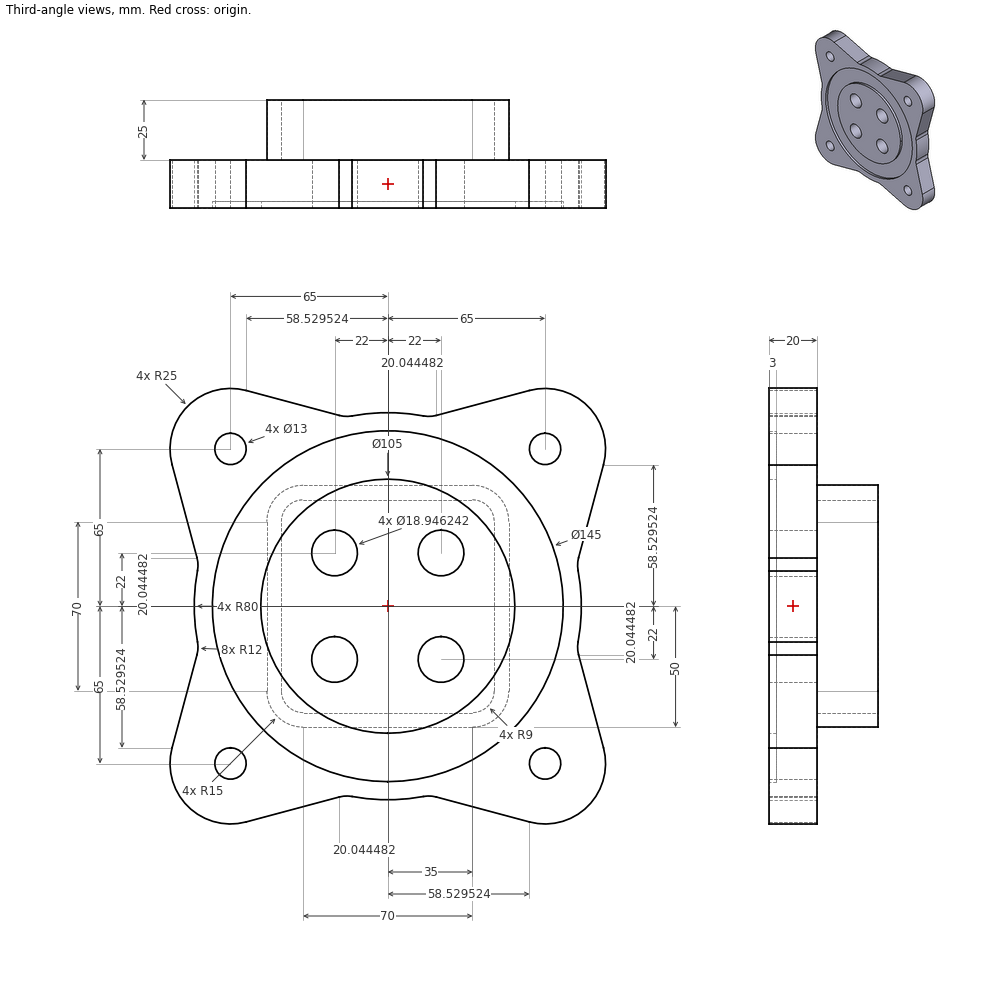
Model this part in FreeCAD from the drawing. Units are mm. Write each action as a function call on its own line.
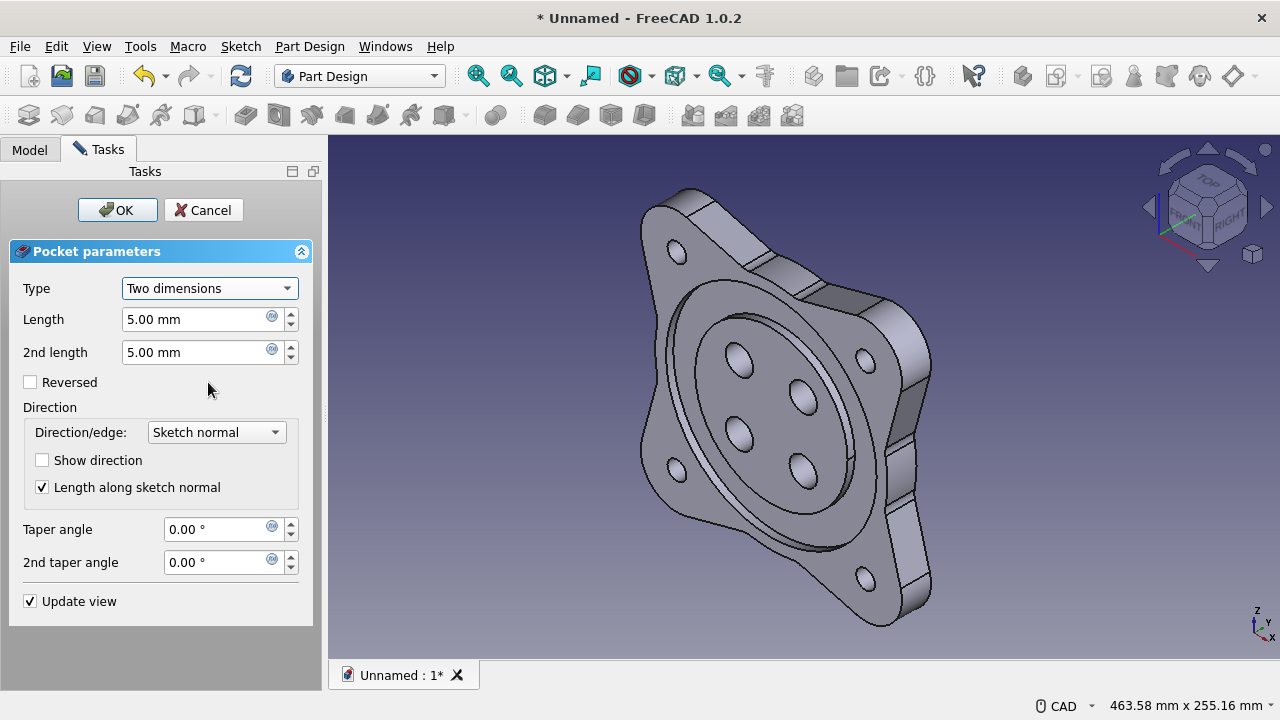
triple_click(204, 320)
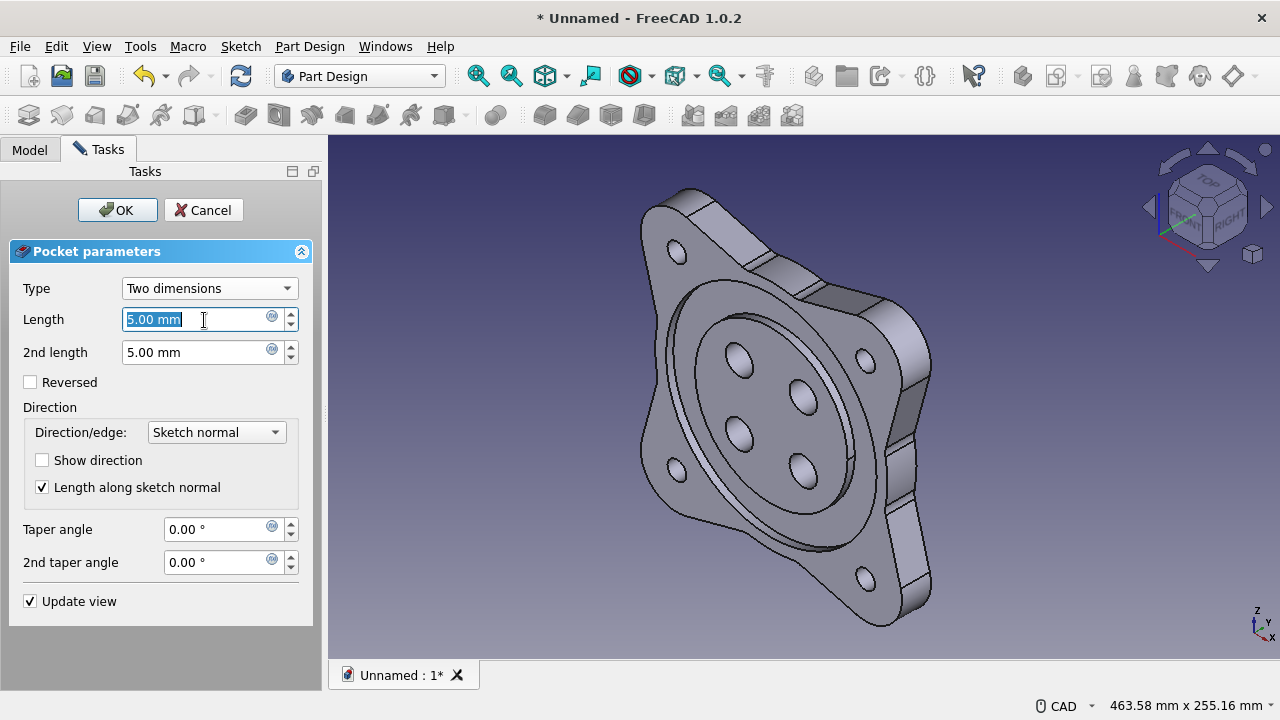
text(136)
key(Tab)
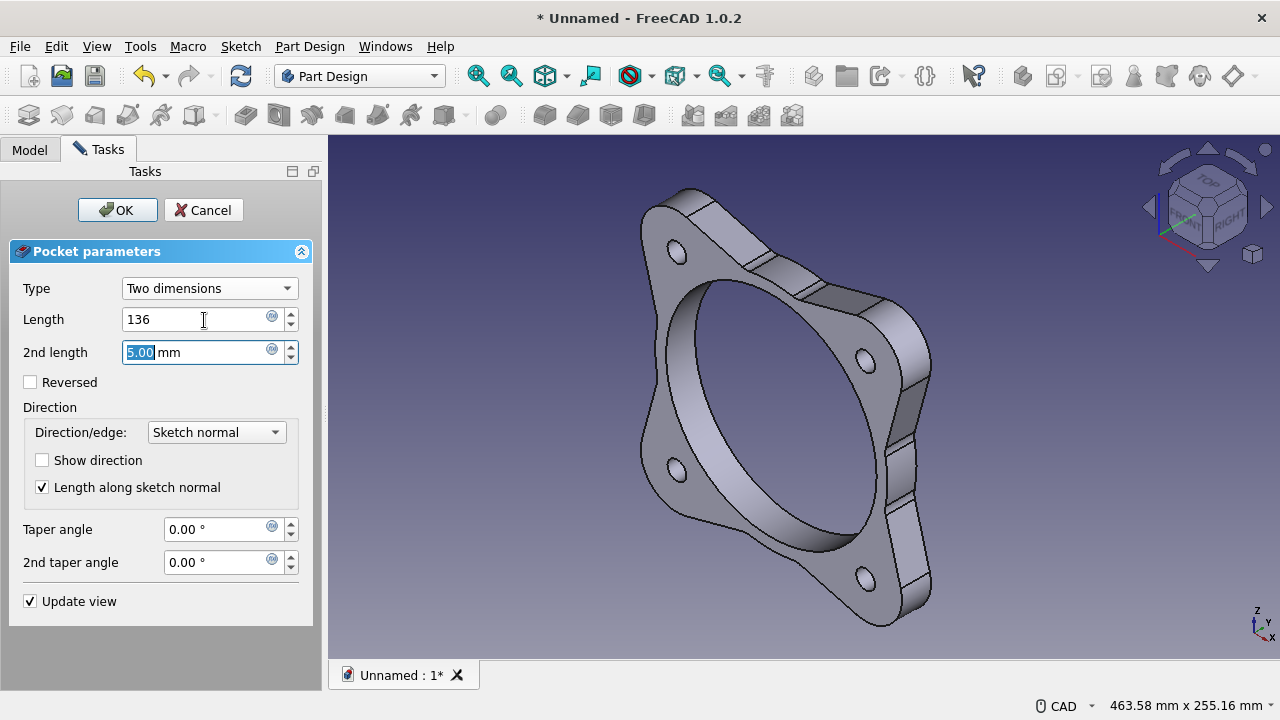
text(3)
key(Tab)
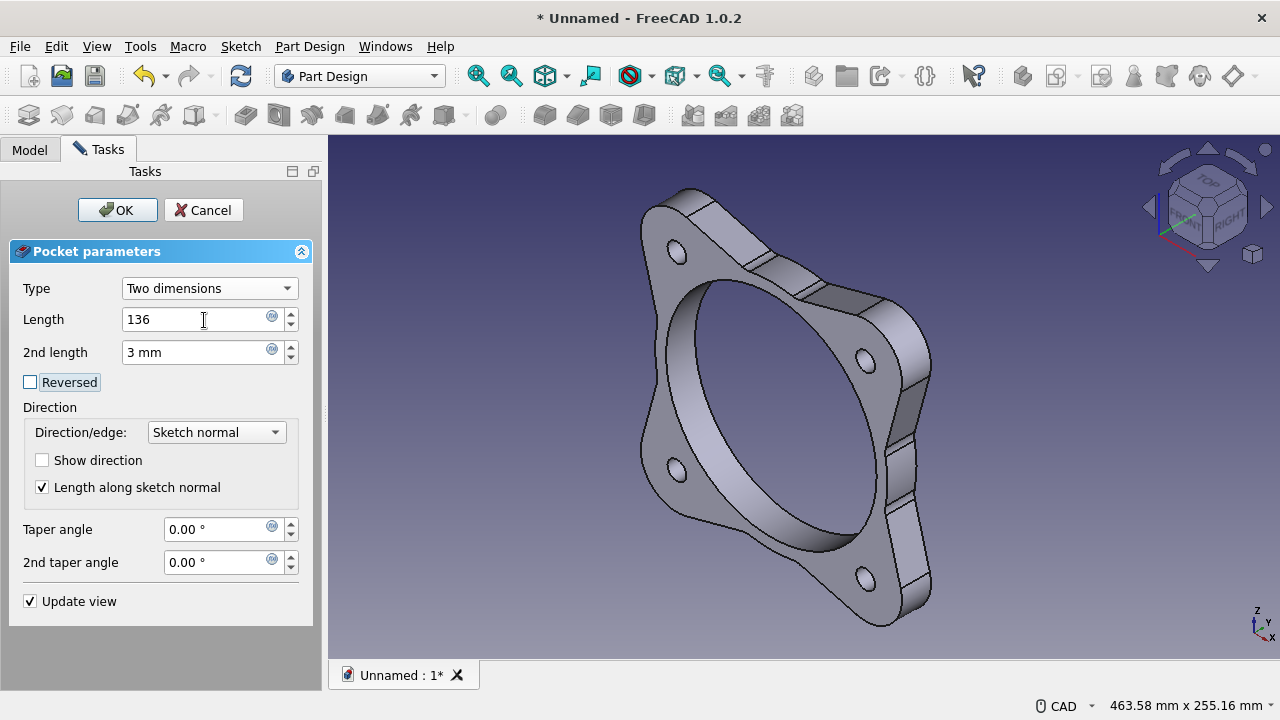
click(31, 382)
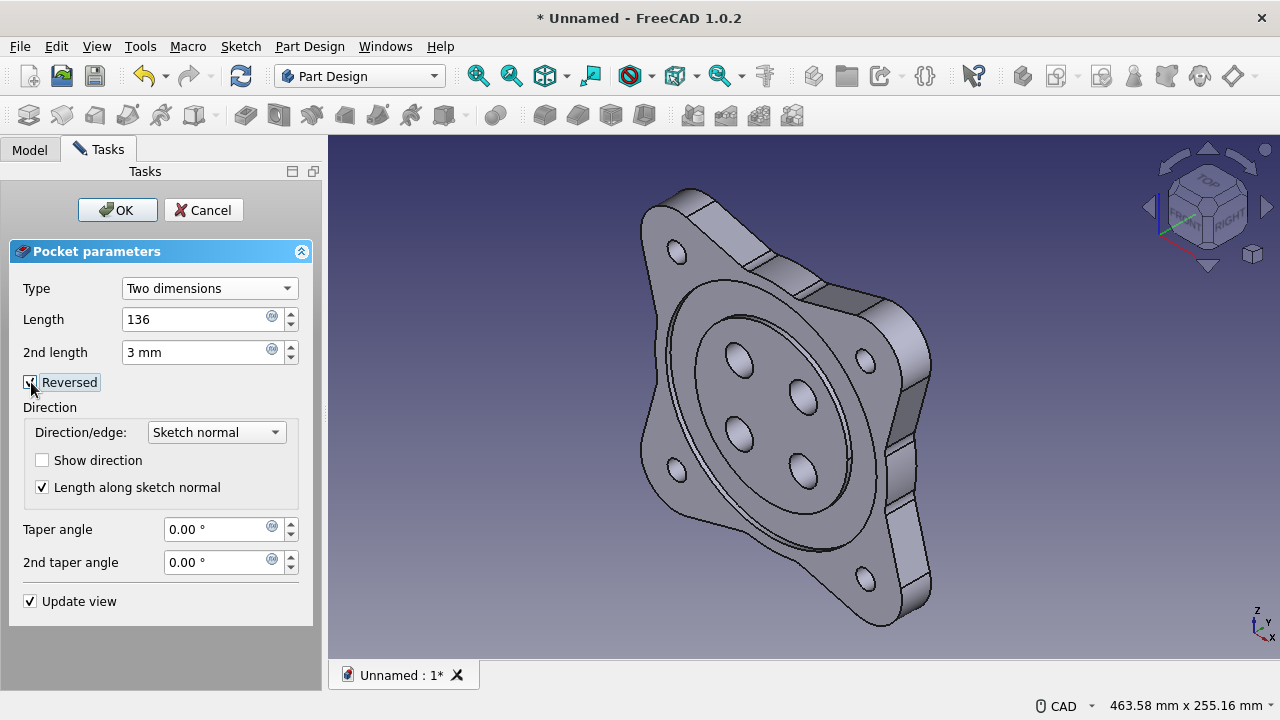
click(118, 210)